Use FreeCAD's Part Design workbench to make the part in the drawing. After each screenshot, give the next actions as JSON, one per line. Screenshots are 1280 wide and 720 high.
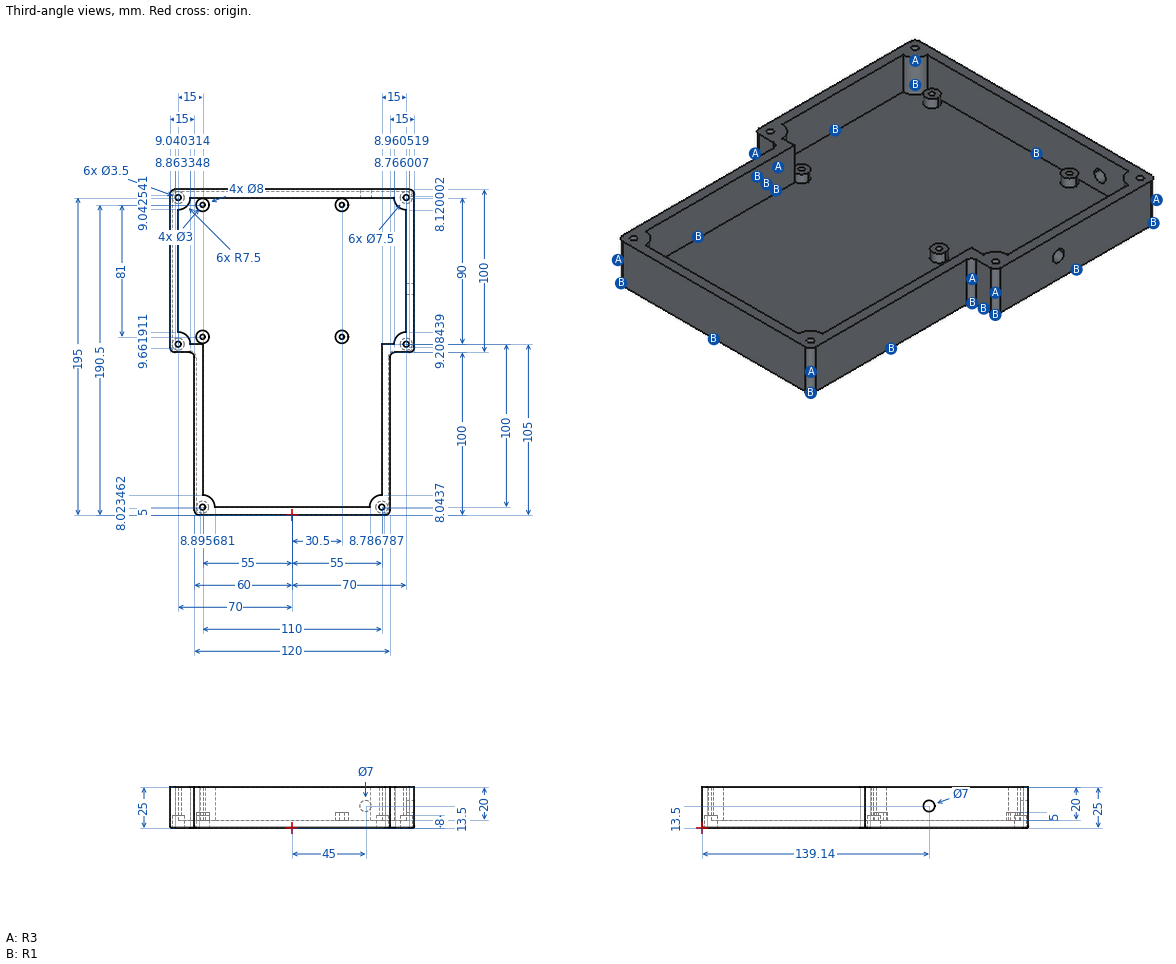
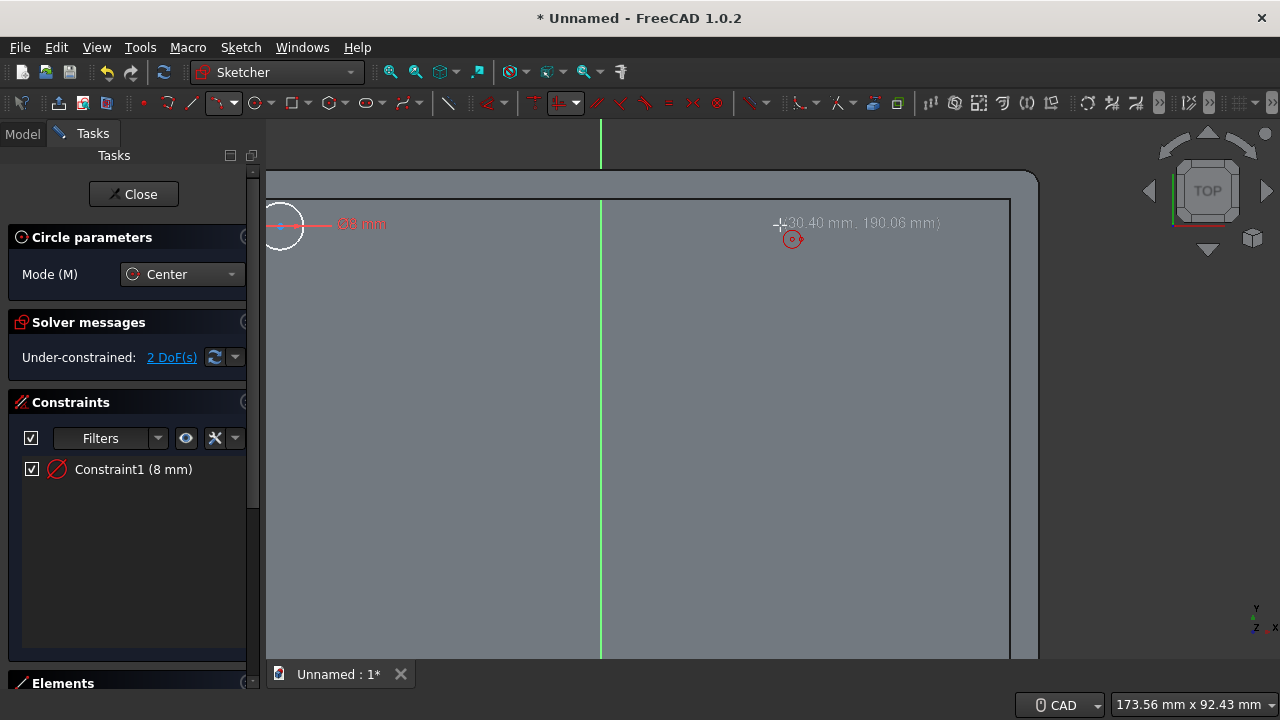
{"action": "left_click", "coordinate": [779, 225]}
{"action": "mouse_move", "coordinate": [796, 209]}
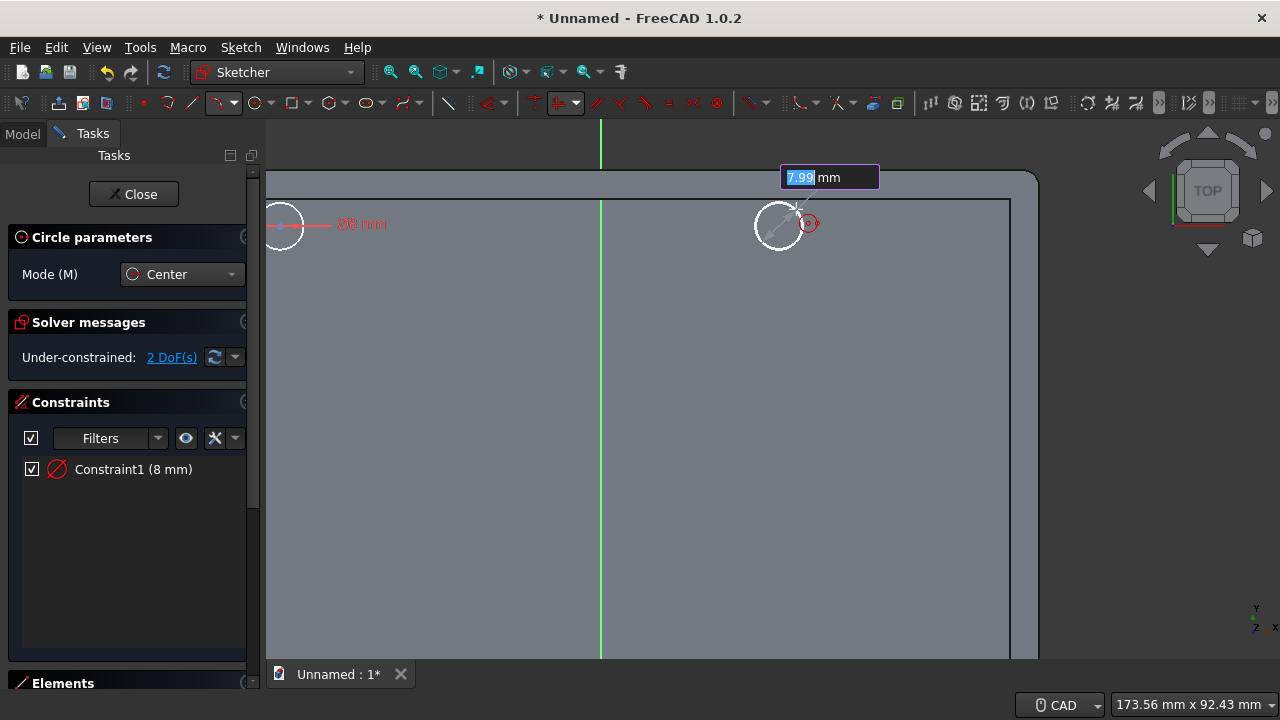
{"action": "type", "text": "8"}
{"action": "key", "text": "Return"}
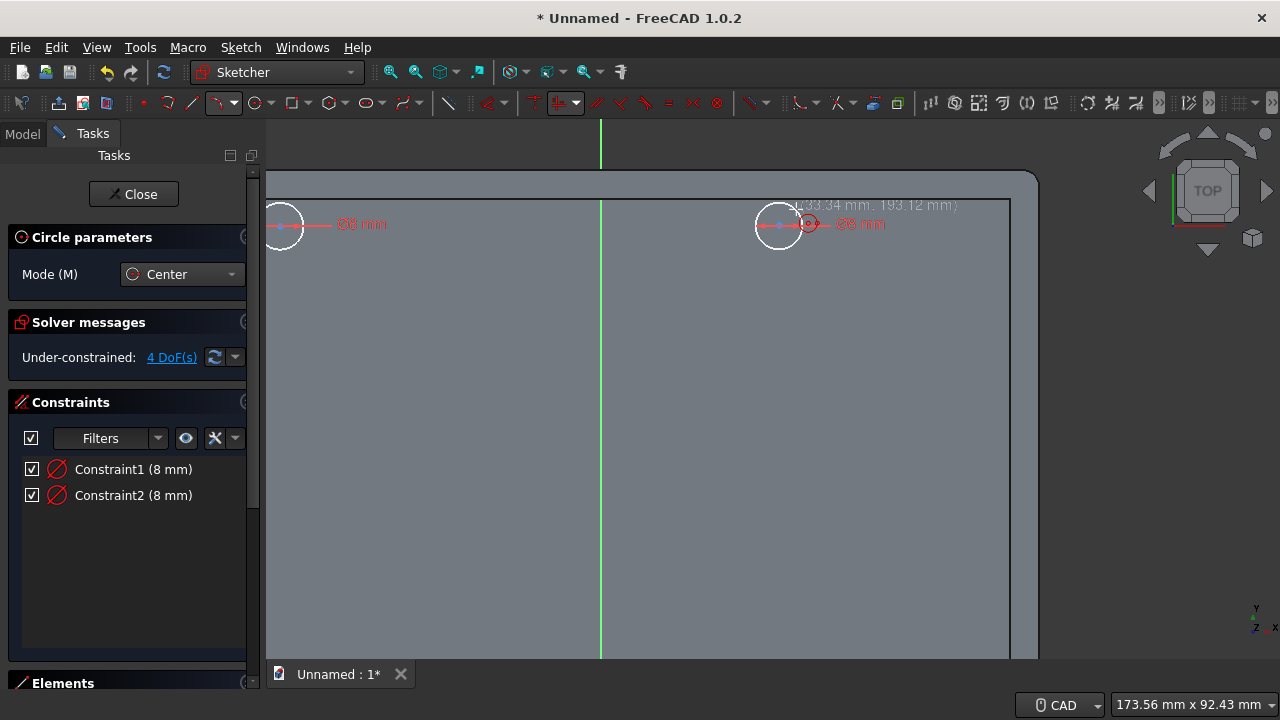
{"action": "scroll", "coordinate": [780, 225], "scroll_direction": "down", "scroll_amount": 6}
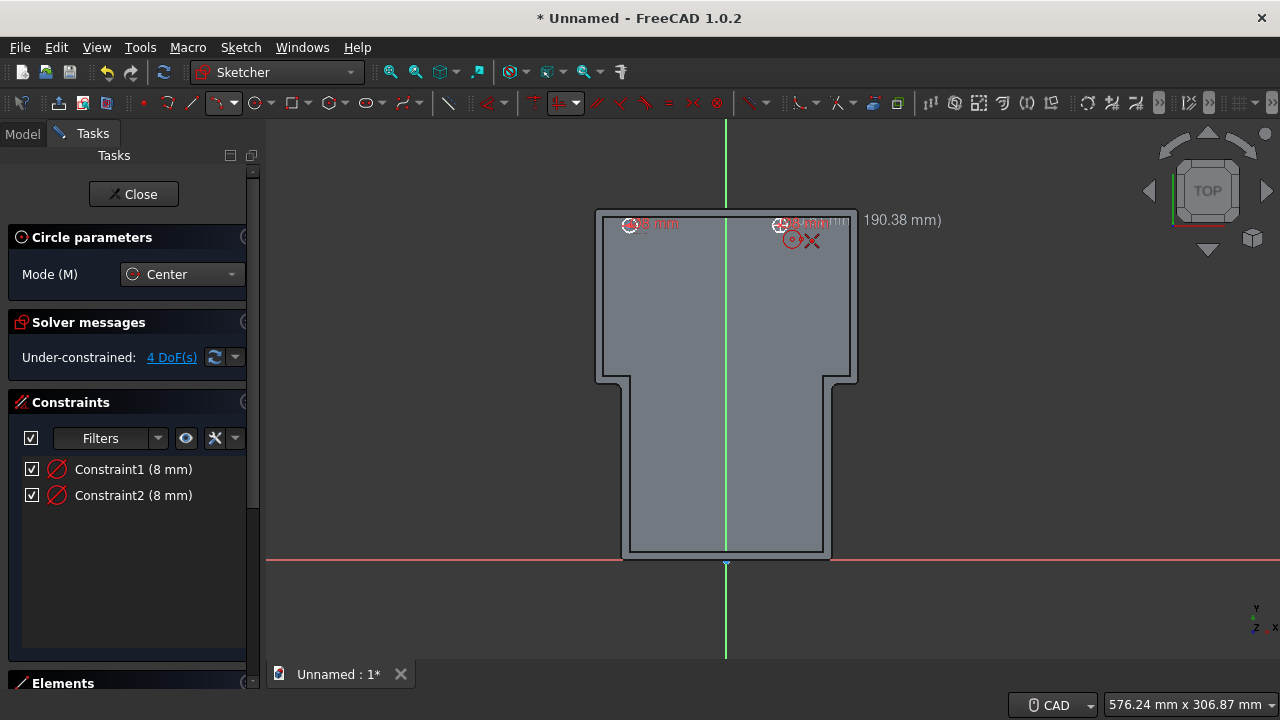
{"action": "scroll", "coordinate": [630, 368], "scroll_direction": "up", "scroll_amount": 6}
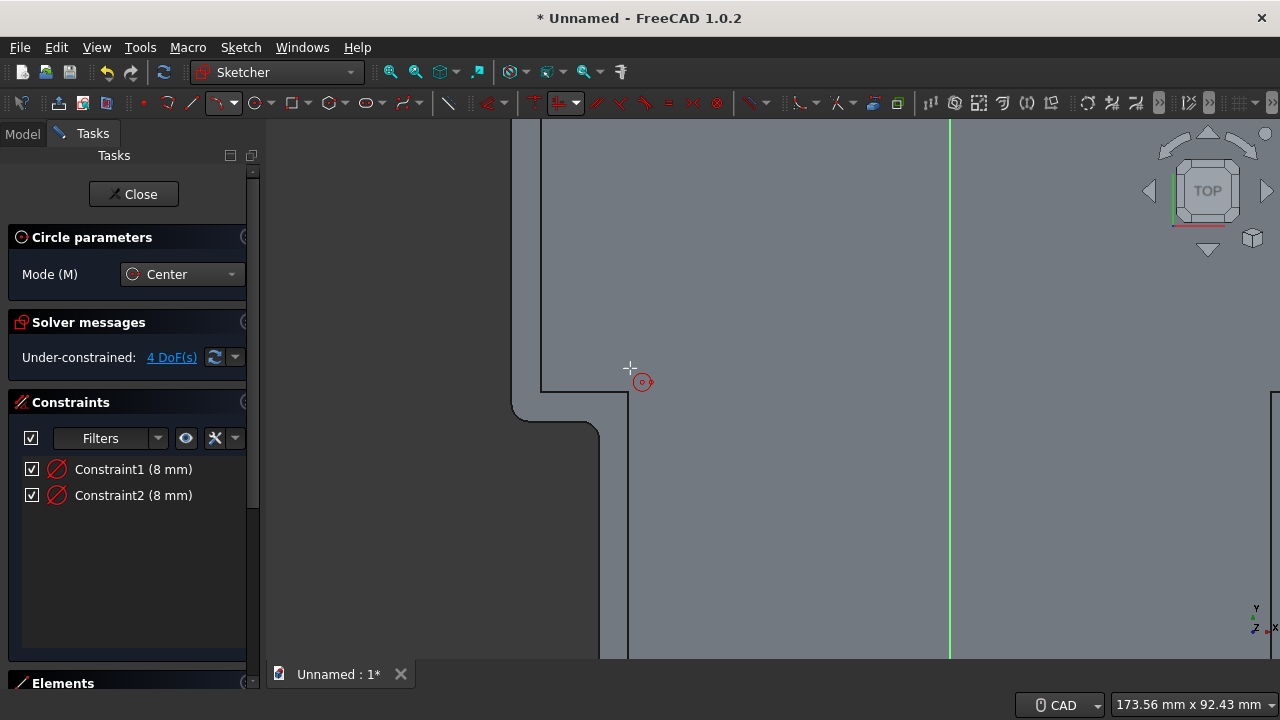
{"action": "left_click", "coordinate": [628, 366]}
{"action": "mouse_move", "coordinate": [645, 350]}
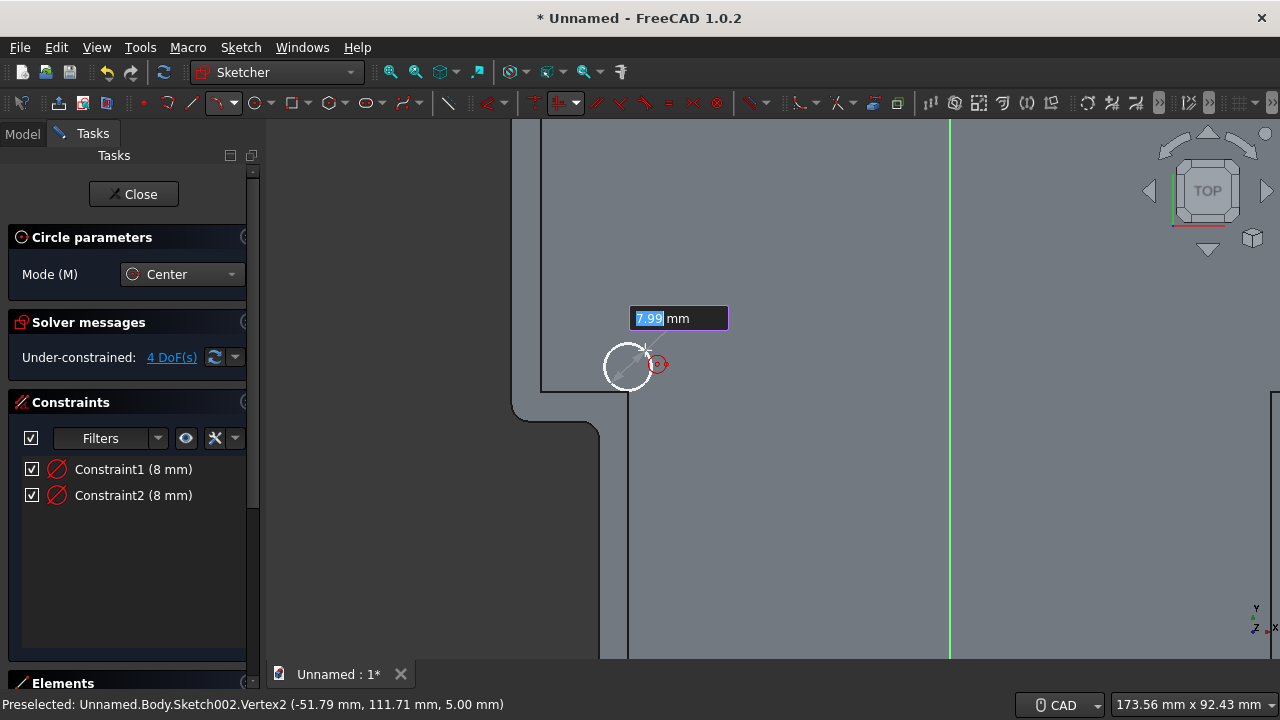
{"action": "type", "text": "8"}
{"action": "key", "text": "Return"}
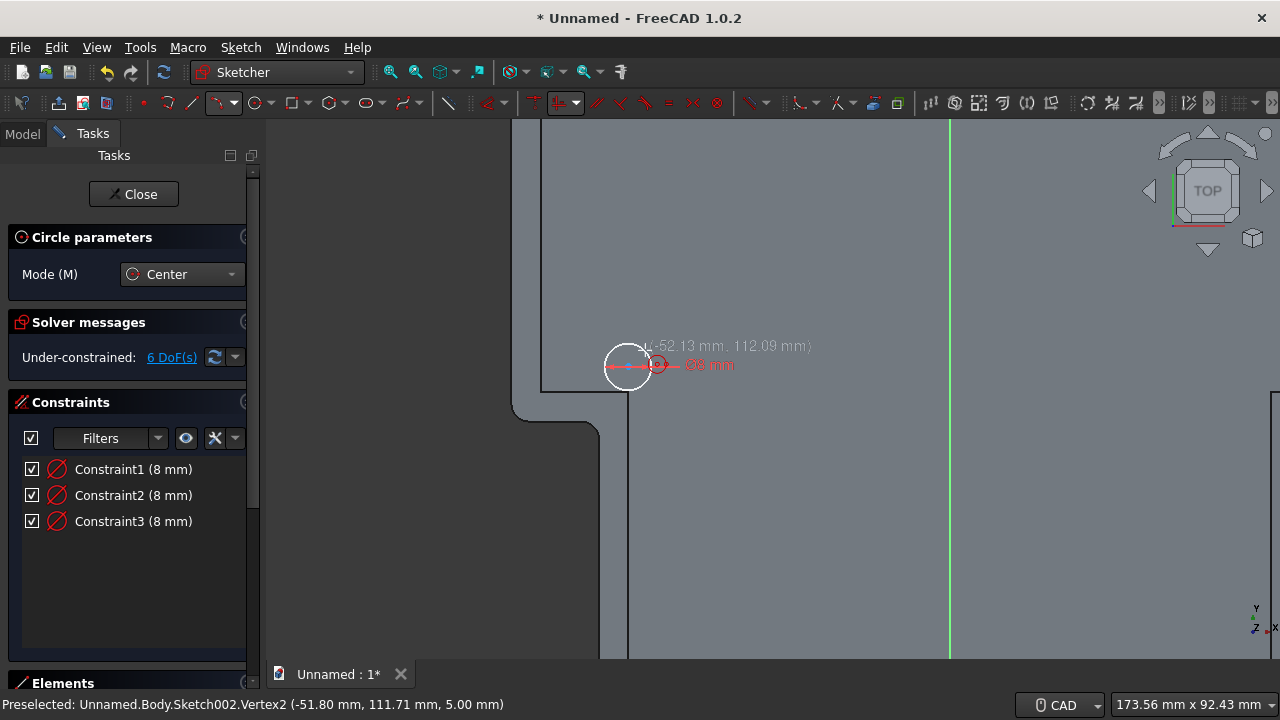
{"action": "scroll", "coordinate": [630, 368], "scroll_direction": "down", "scroll_amount": 6}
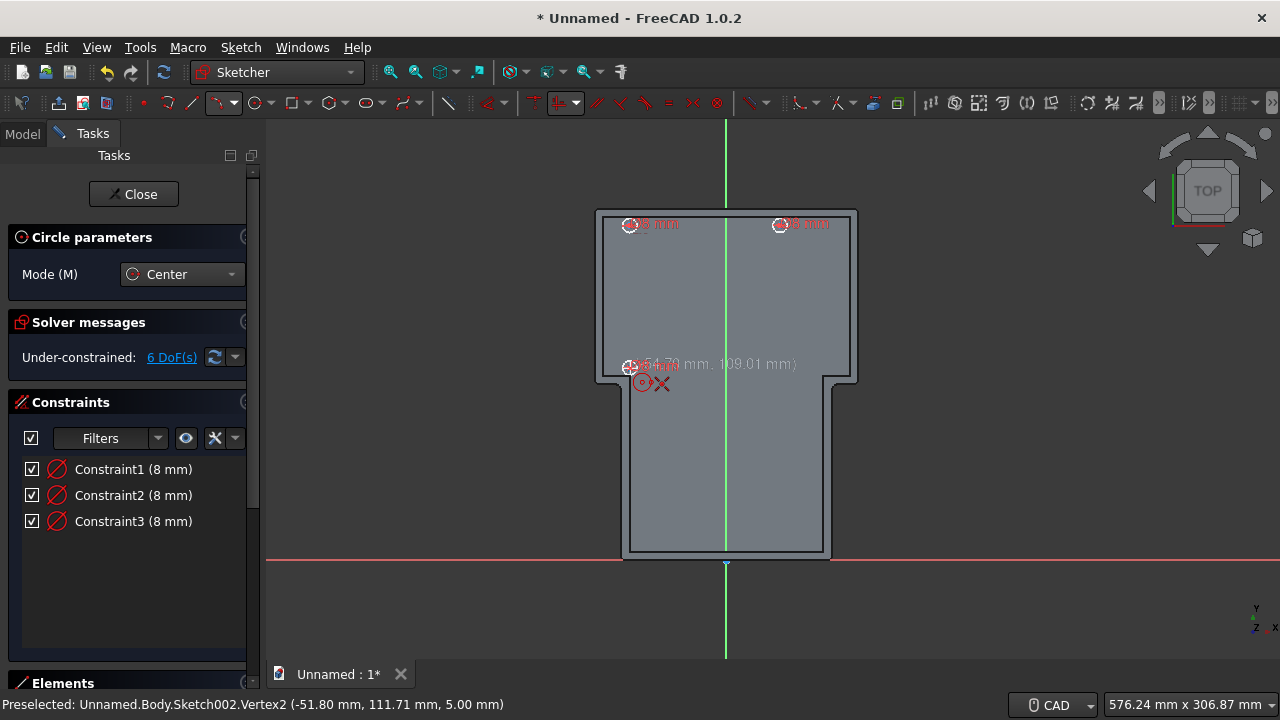
{"action": "scroll", "coordinate": [780, 368], "scroll_direction": "up", "scroll_amount": 6}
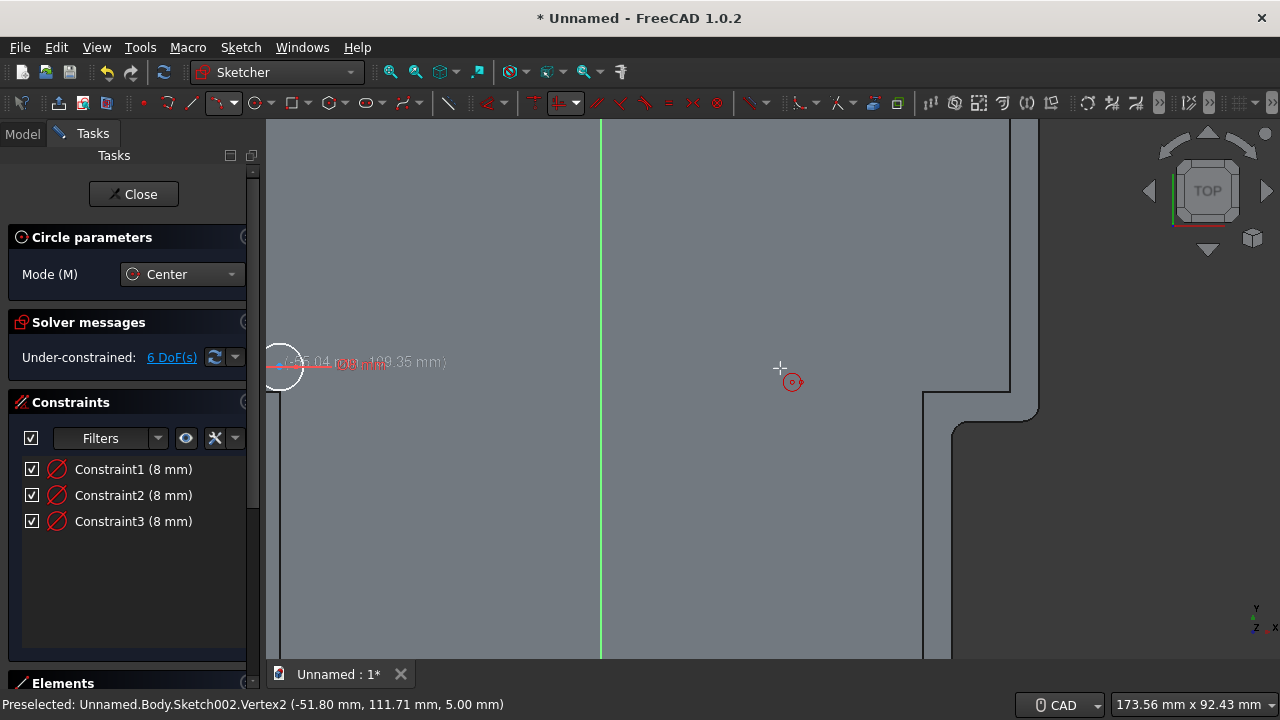
{"action": "left_click", "coordinate": [779, 366]}
{"action": "mouse_move", "coordinate": [796, 350]}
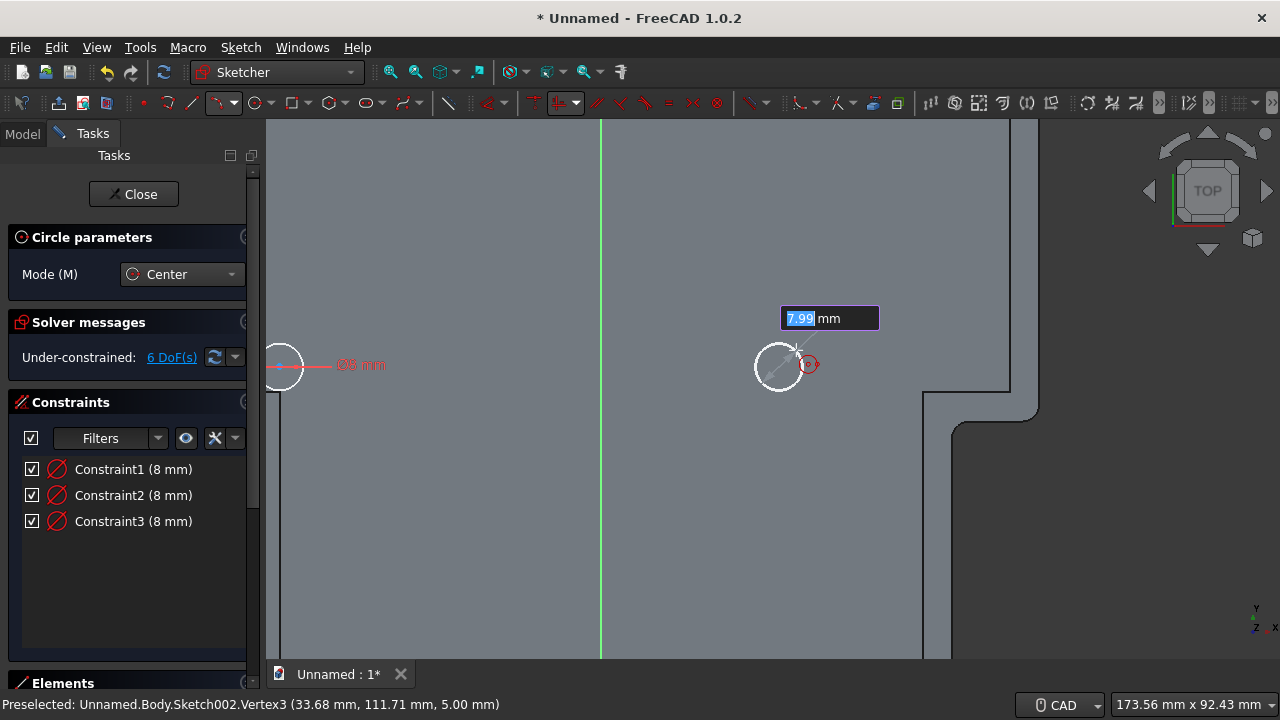
{"action": "type", "text": "8"}
{"action": "key", "text": "Return"}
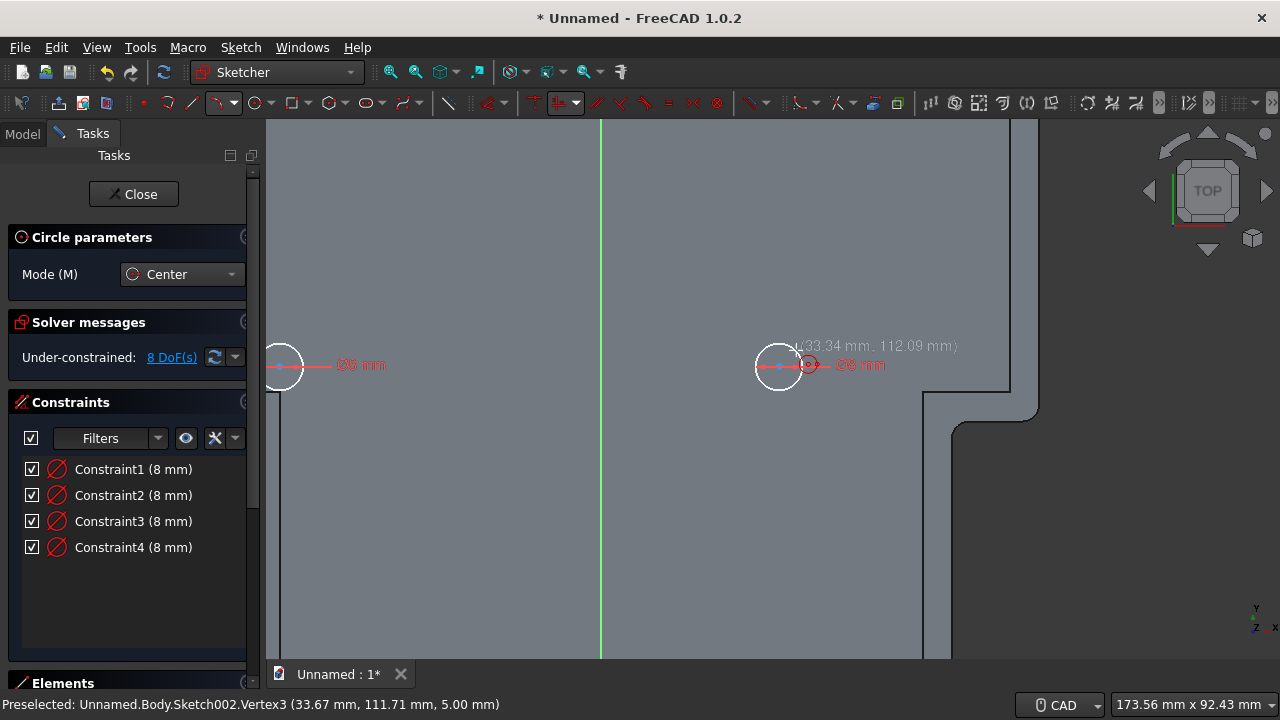
{"action": "scroll", "coordinate": [780, 368], "scroll_direction": "down", "scroll_amount": 6}